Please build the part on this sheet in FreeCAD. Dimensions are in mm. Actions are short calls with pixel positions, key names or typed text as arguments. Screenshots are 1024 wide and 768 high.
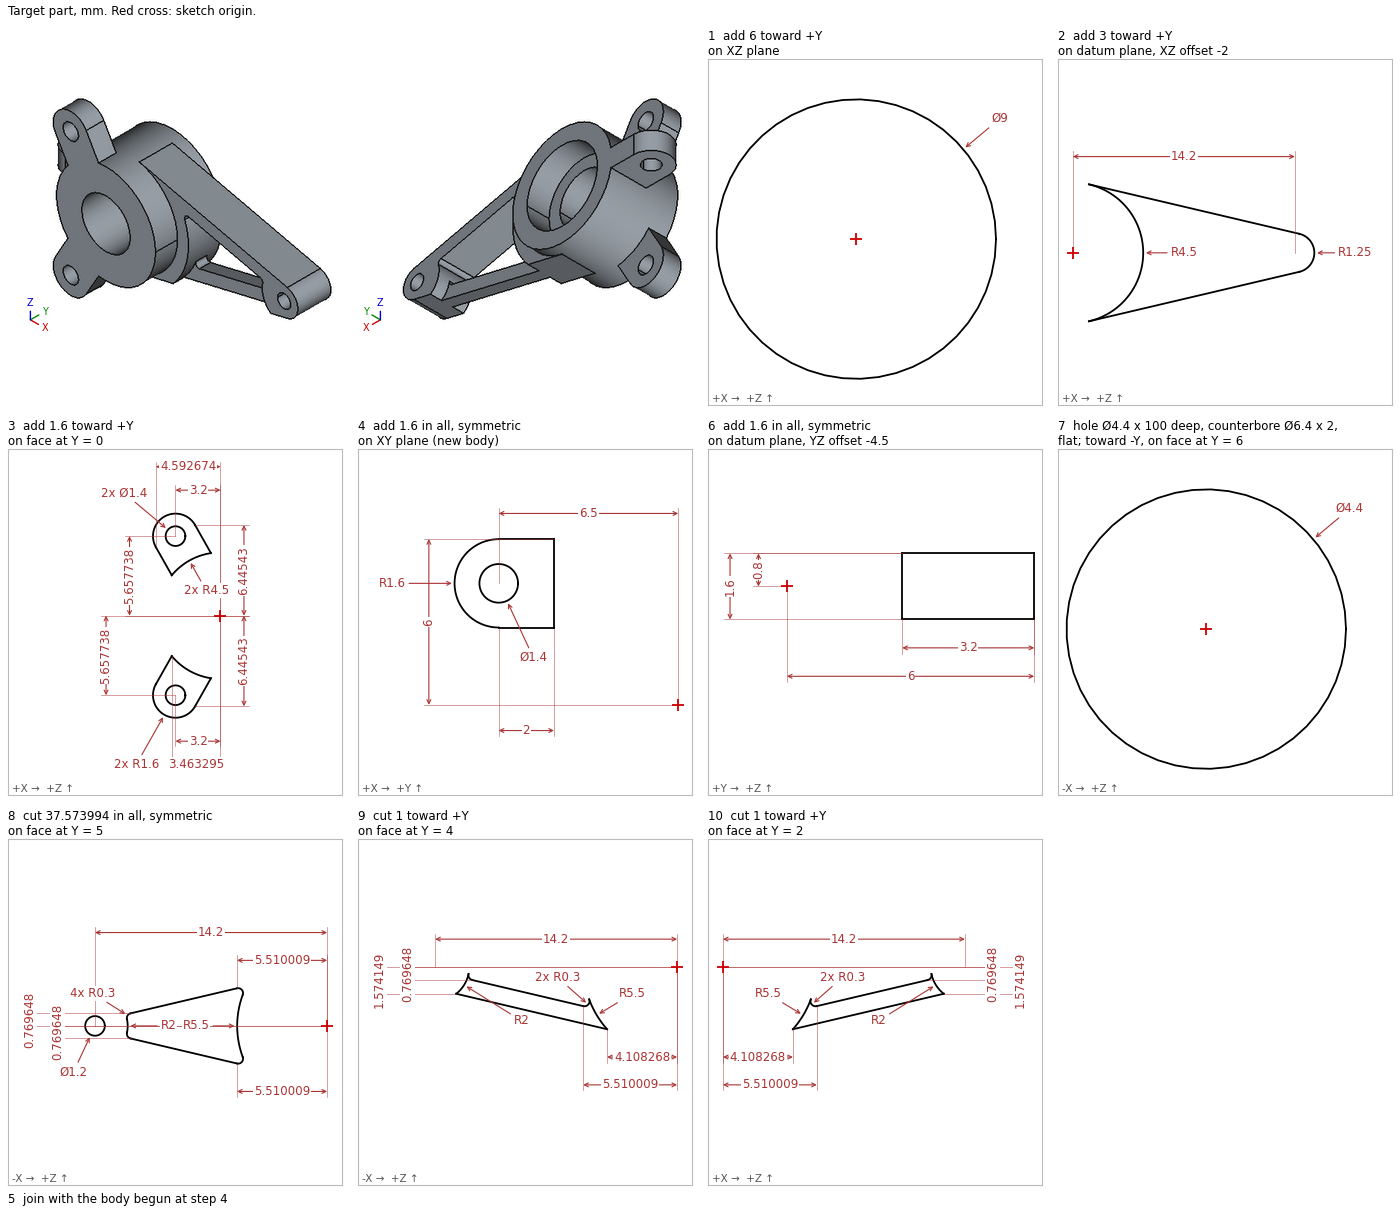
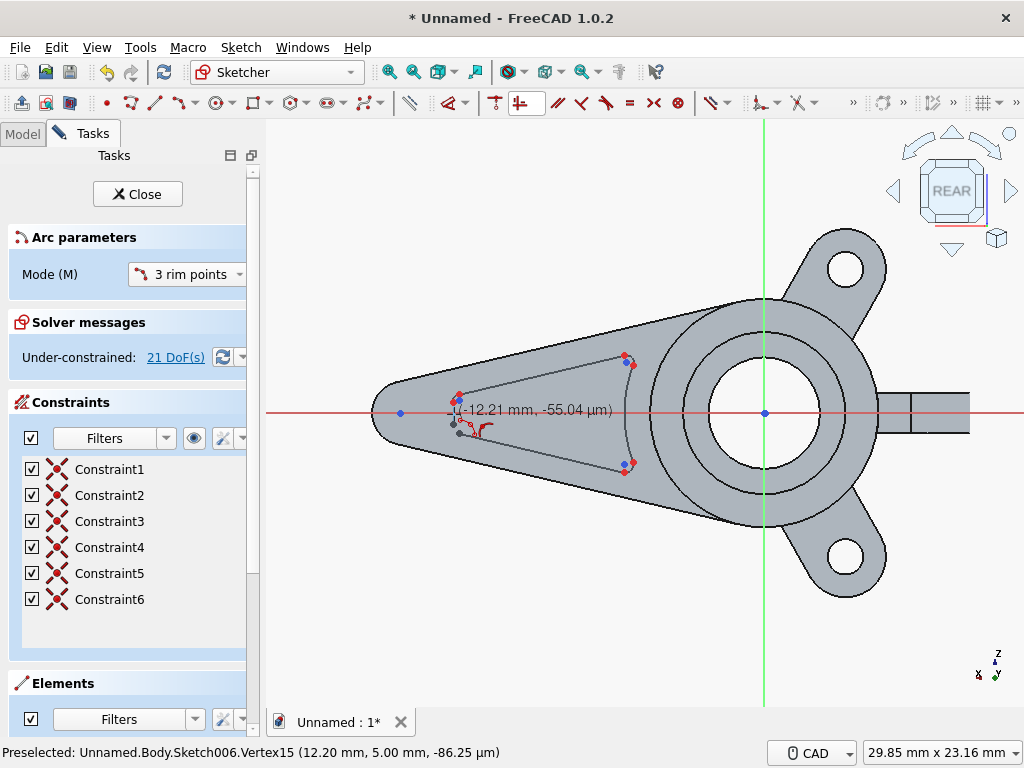
scroll(453, 424, up, 3)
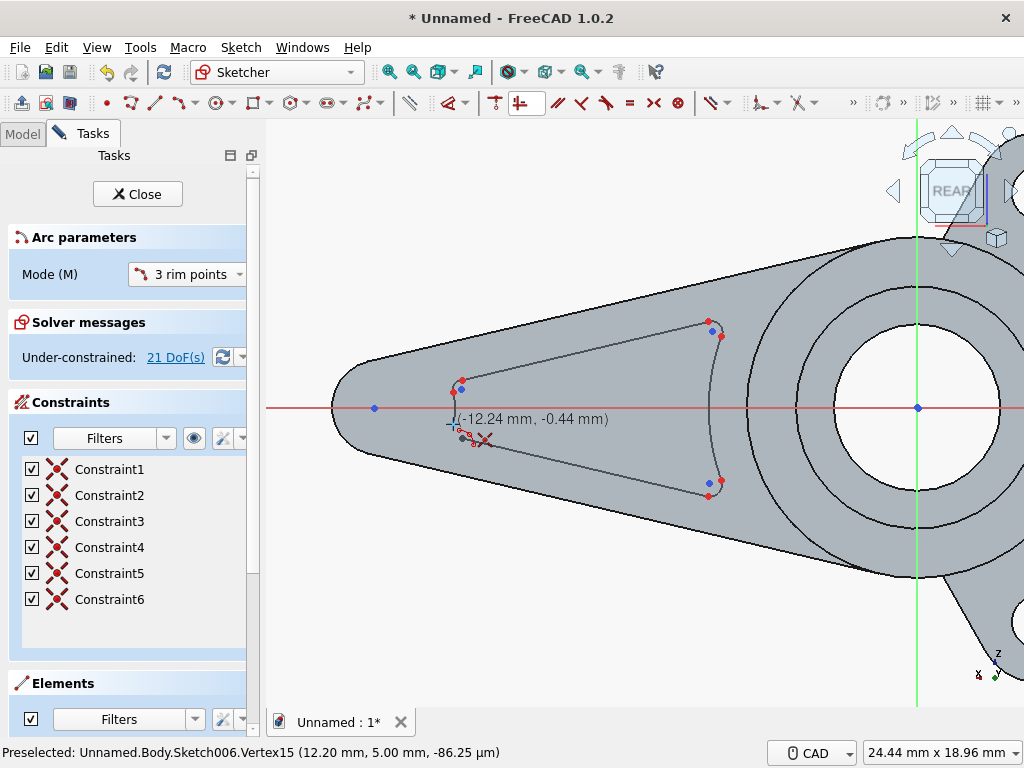
click(453, 424)
click(465, 442)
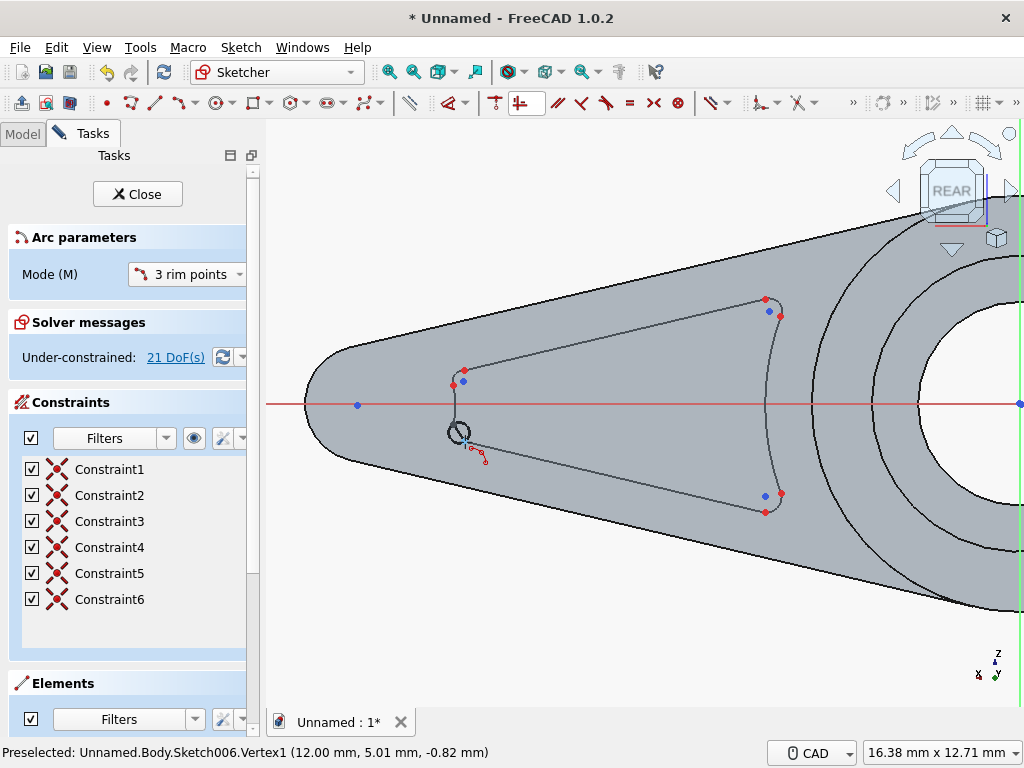
scroll(455, 433, up, 7)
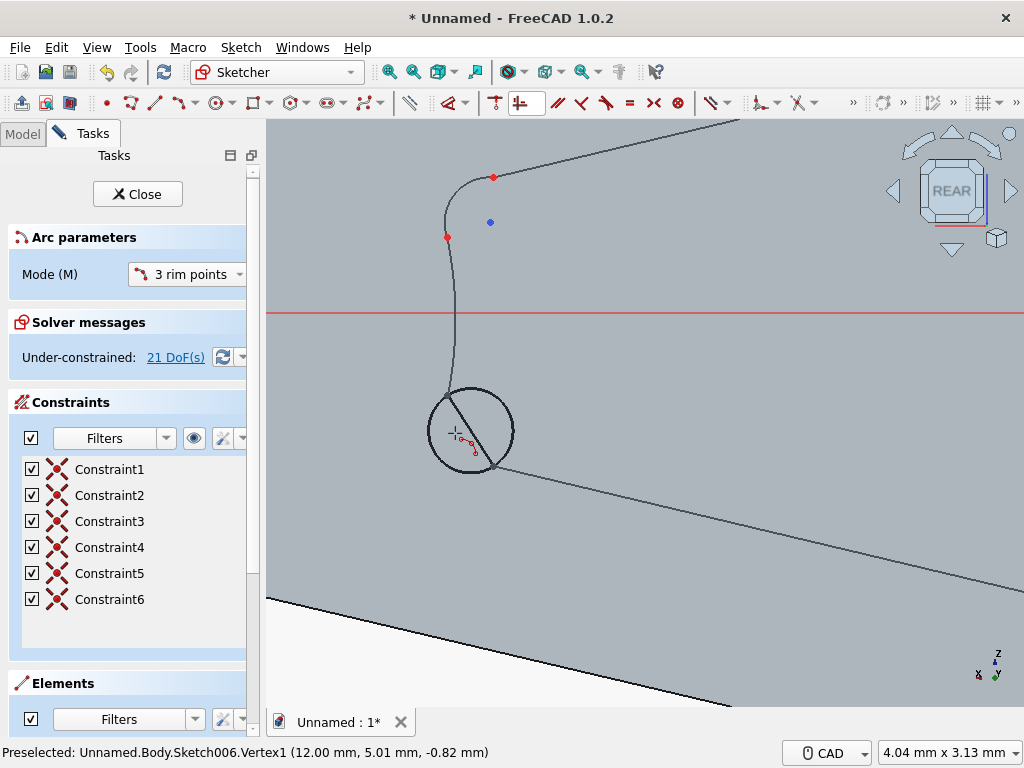
click(455, 433)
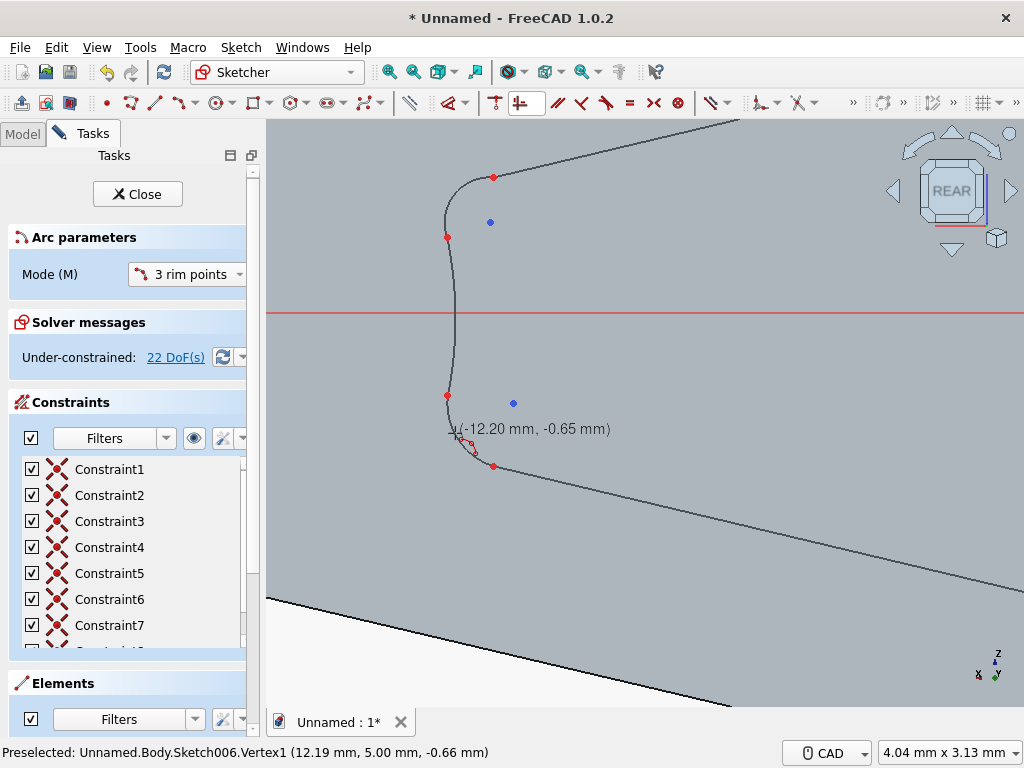
click(216, 104)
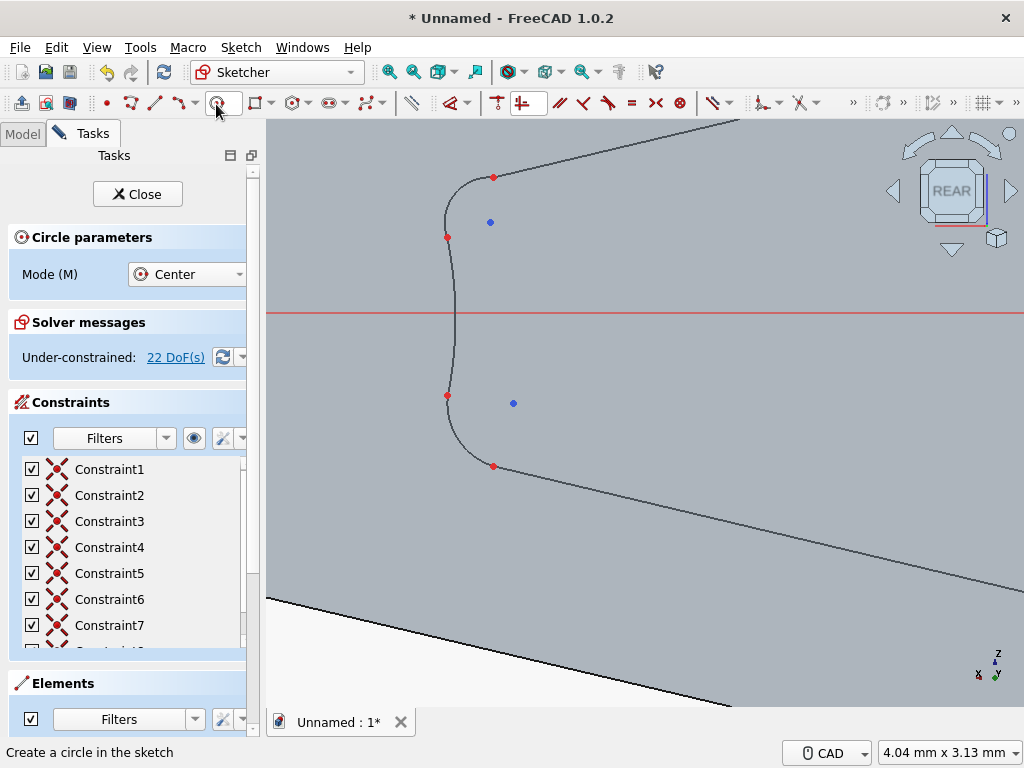
scroll(454, 429, down, 10)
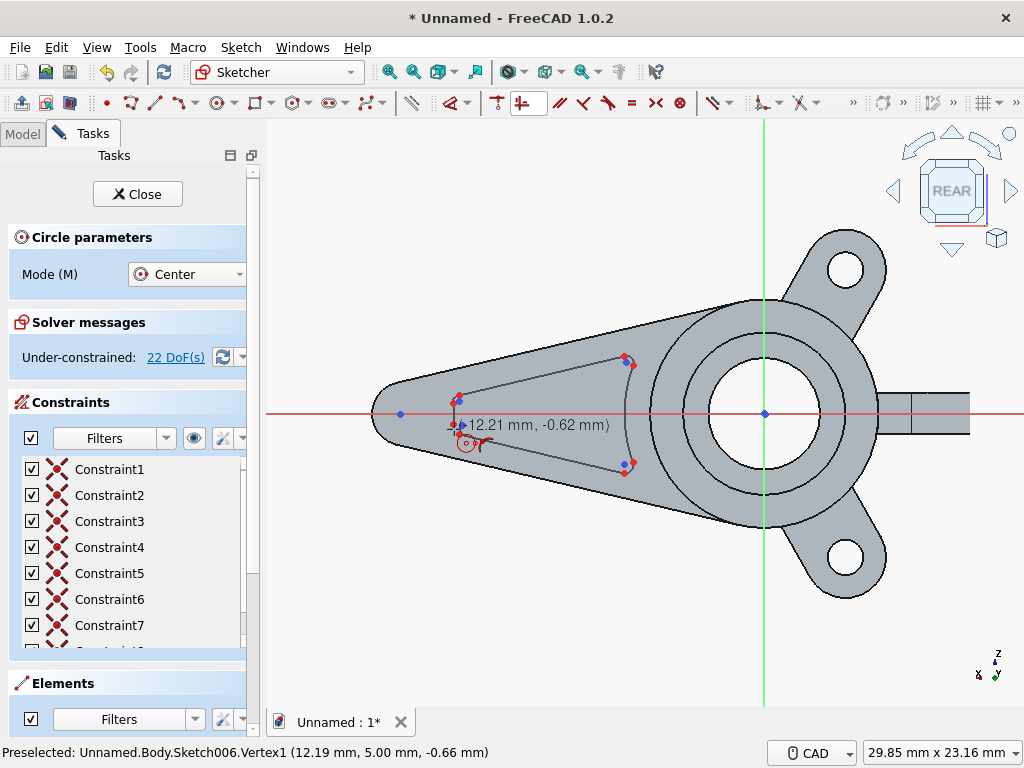
scroll(404, 414, up, 2)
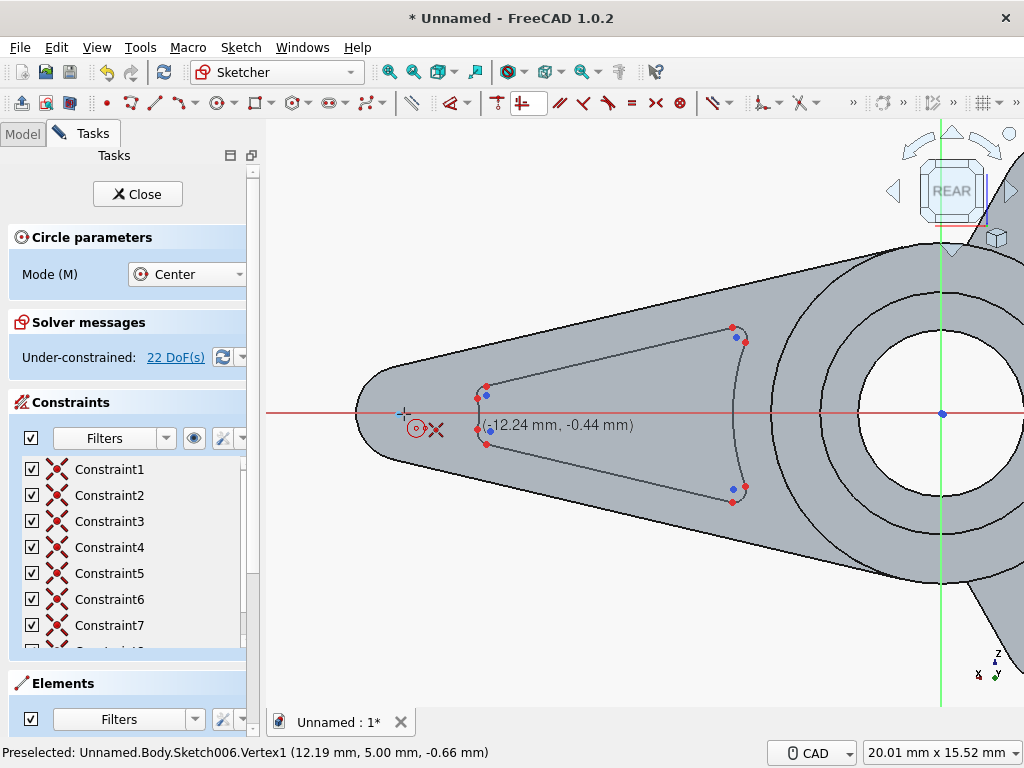
click(403, 413)
click(419, 397)
key(Escape)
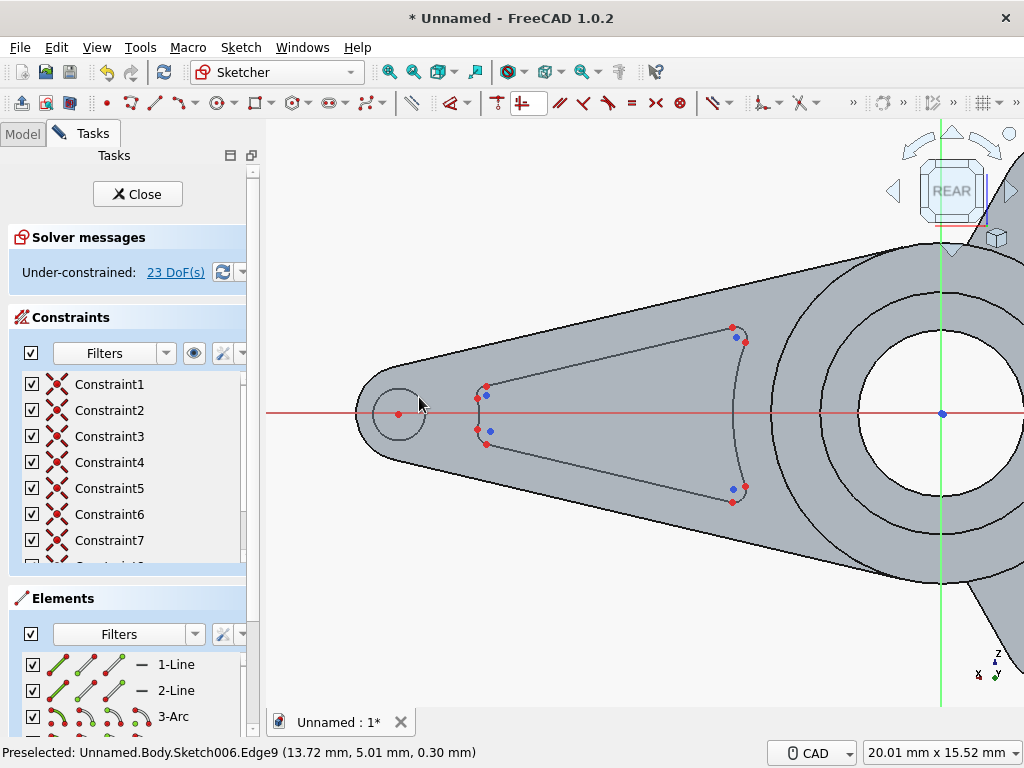
click(561, 462)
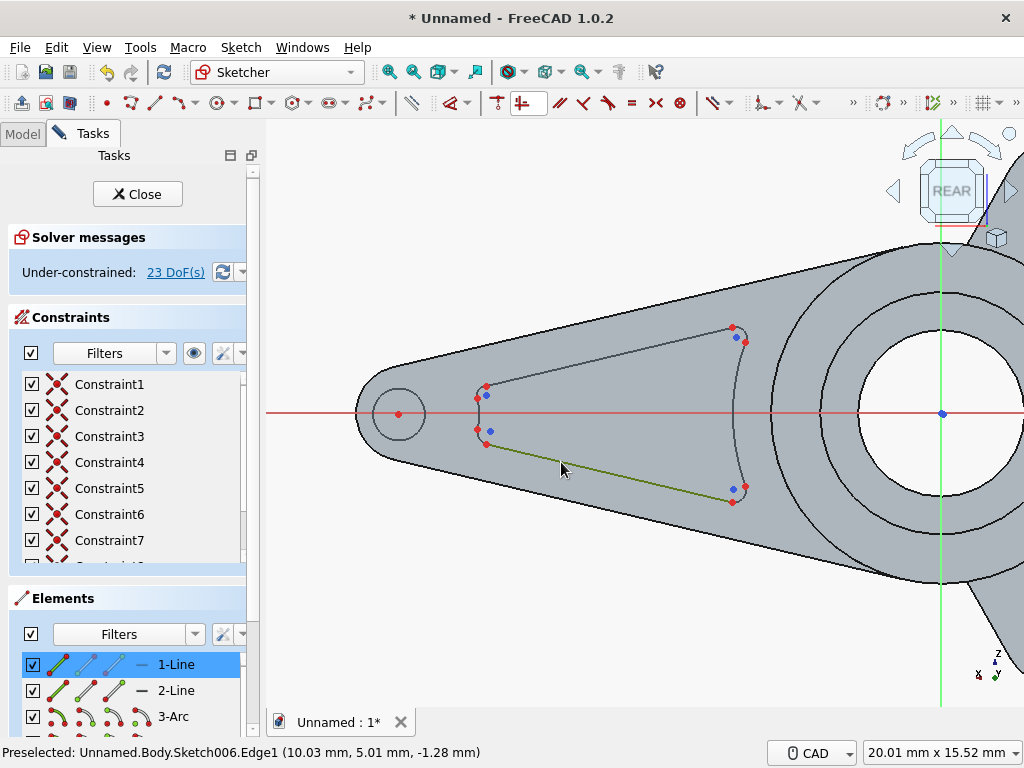
click(743, 498)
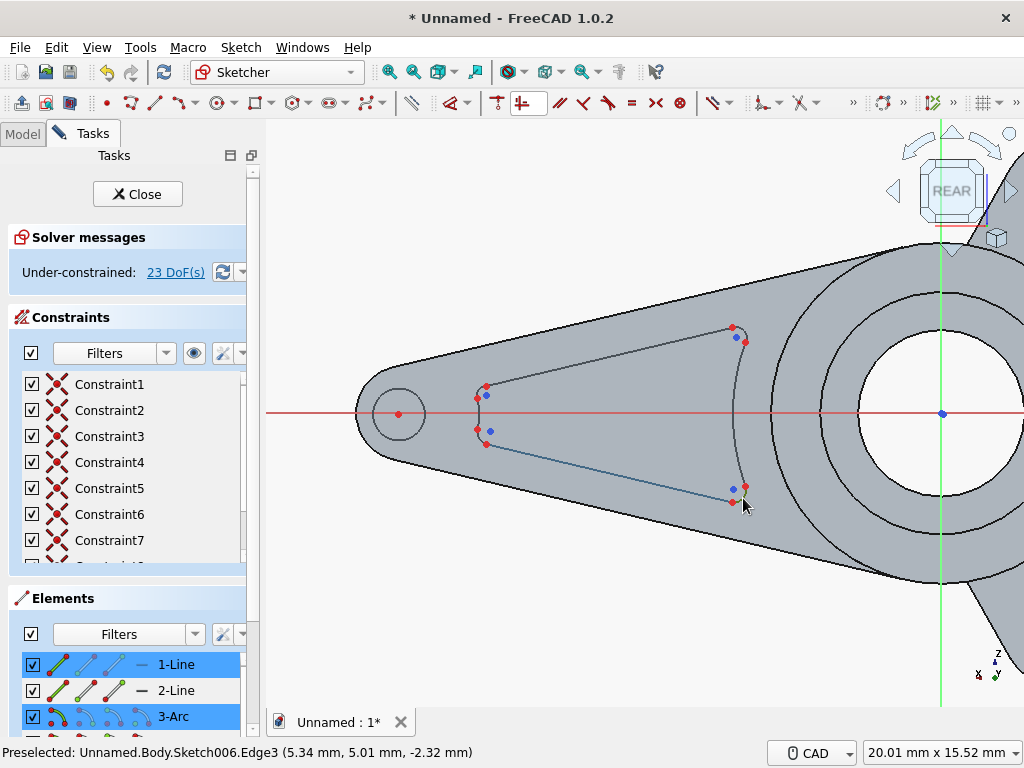
key(t)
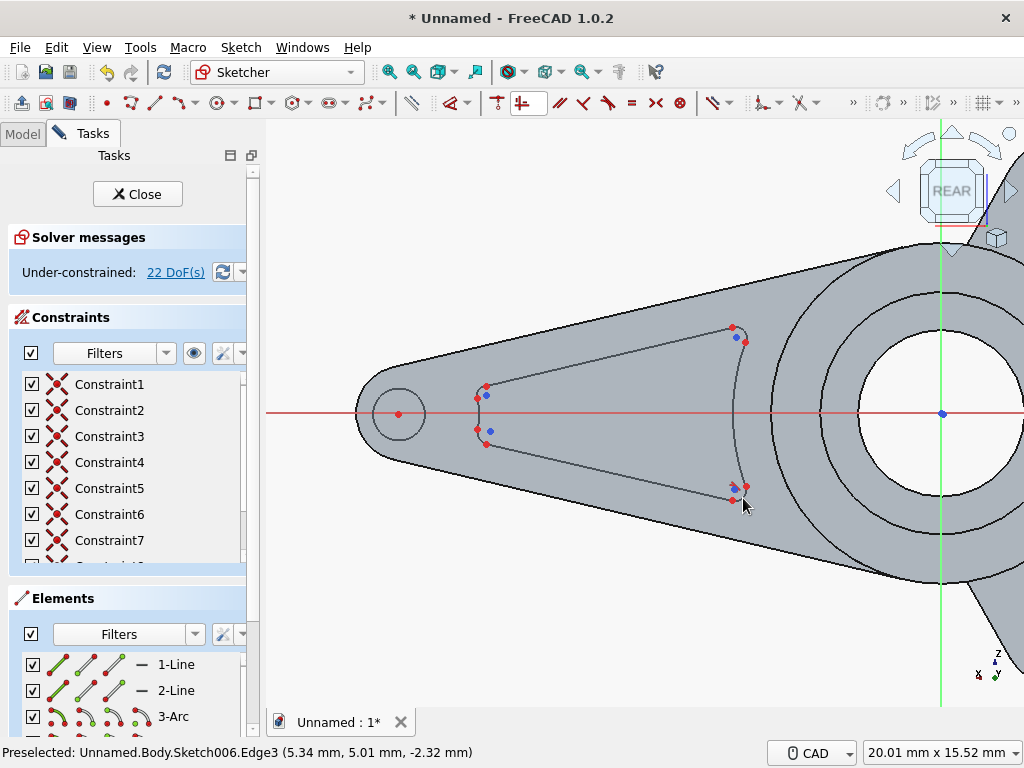
click(560, 461)